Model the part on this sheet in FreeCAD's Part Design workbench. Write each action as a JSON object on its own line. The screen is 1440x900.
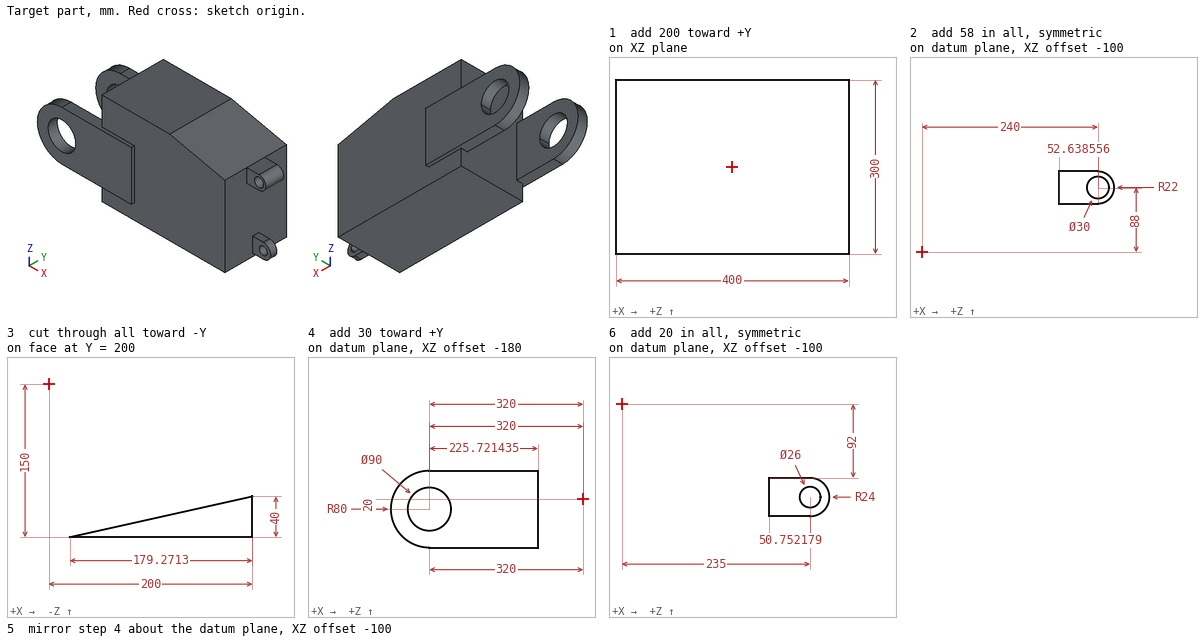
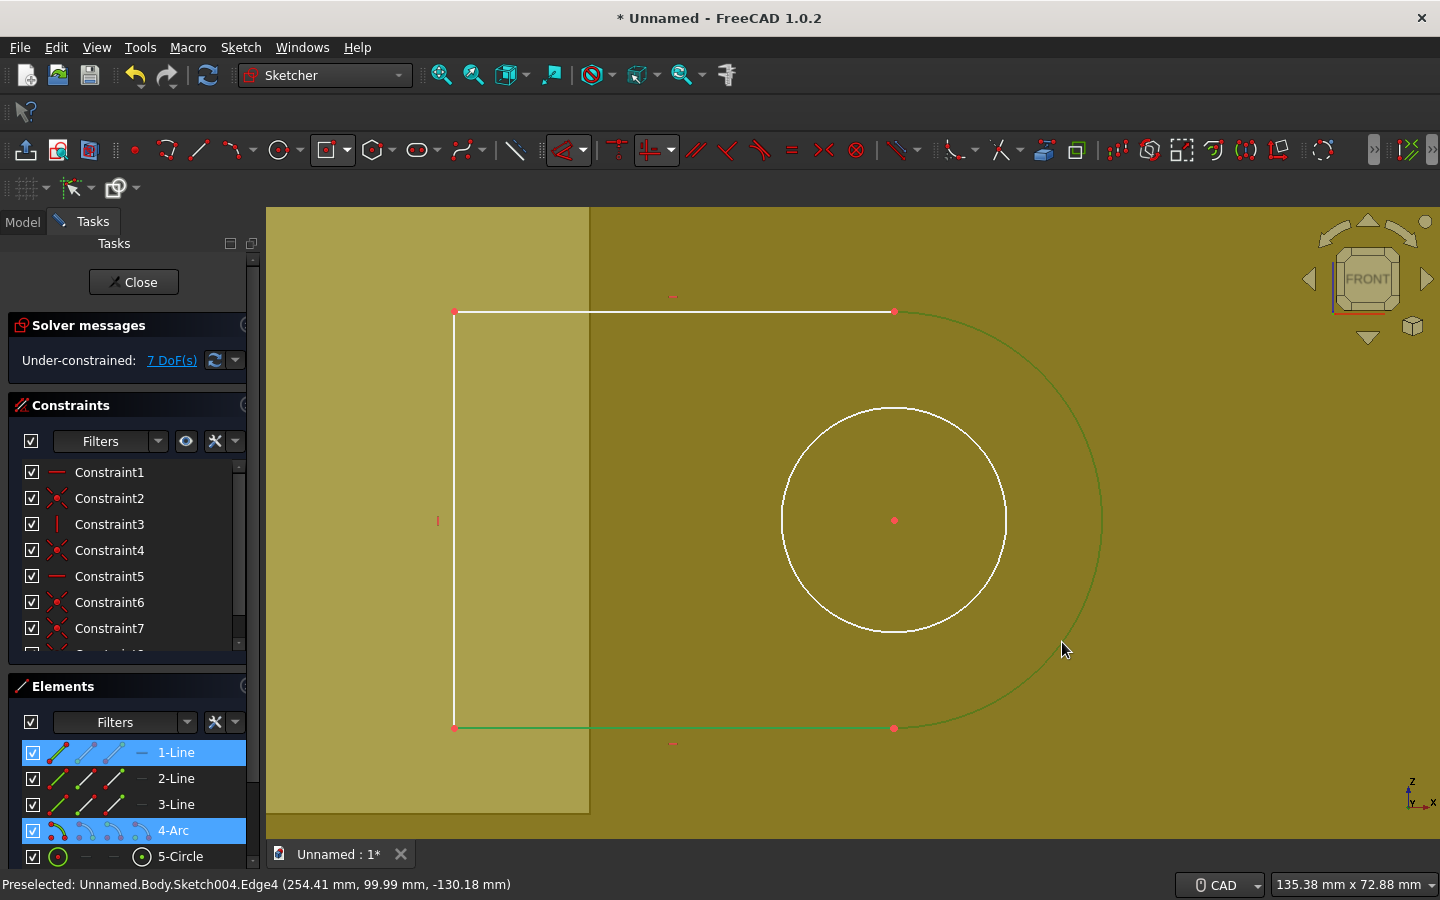
{"action": "left_click", "coordinate": [760, 150]}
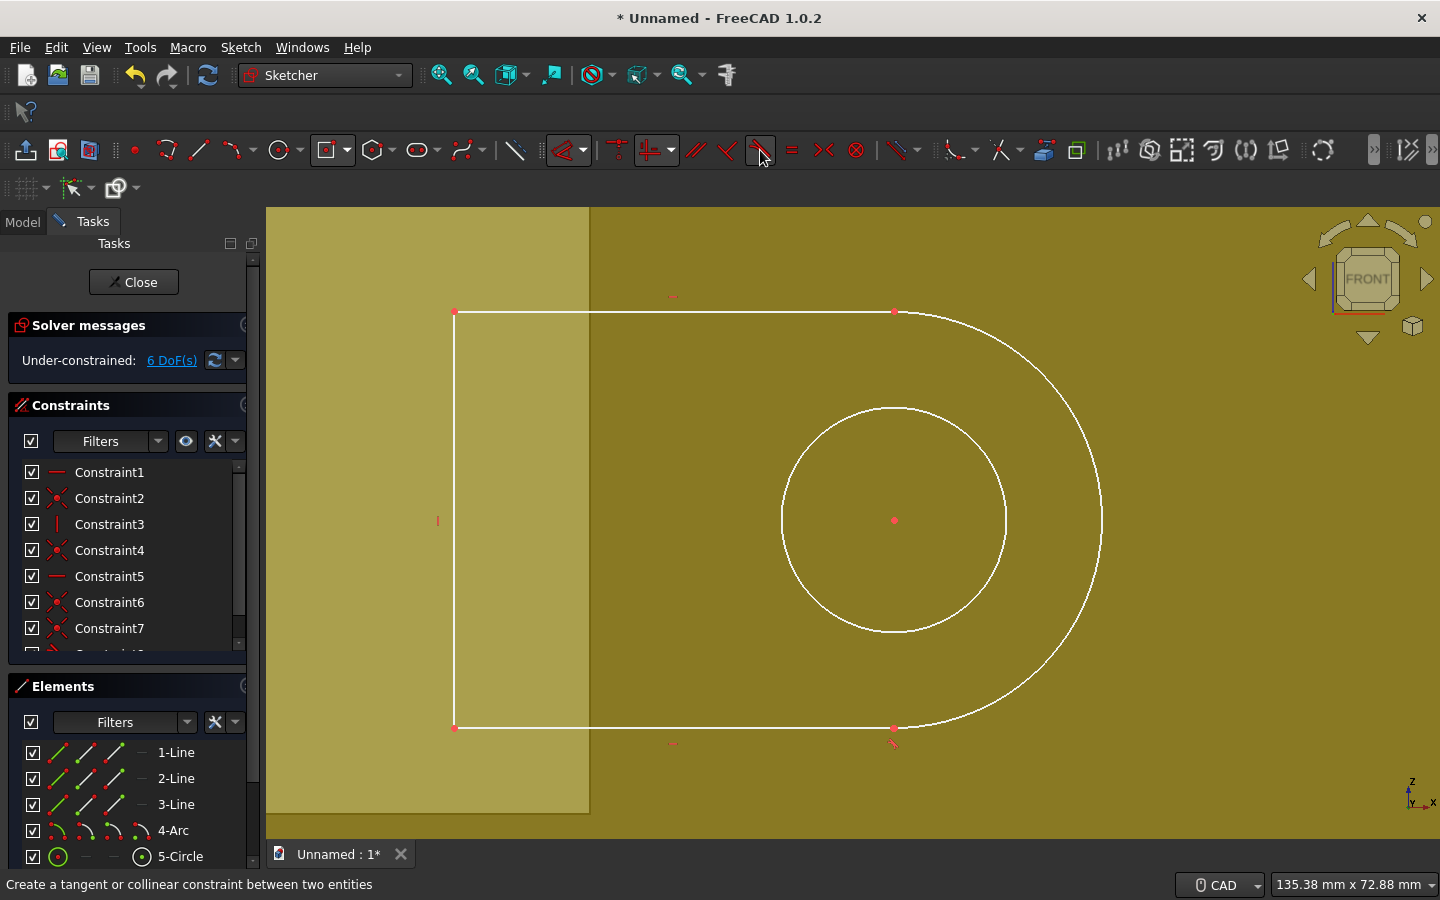
{"action": "left_click", "coordinate": [586, 312]}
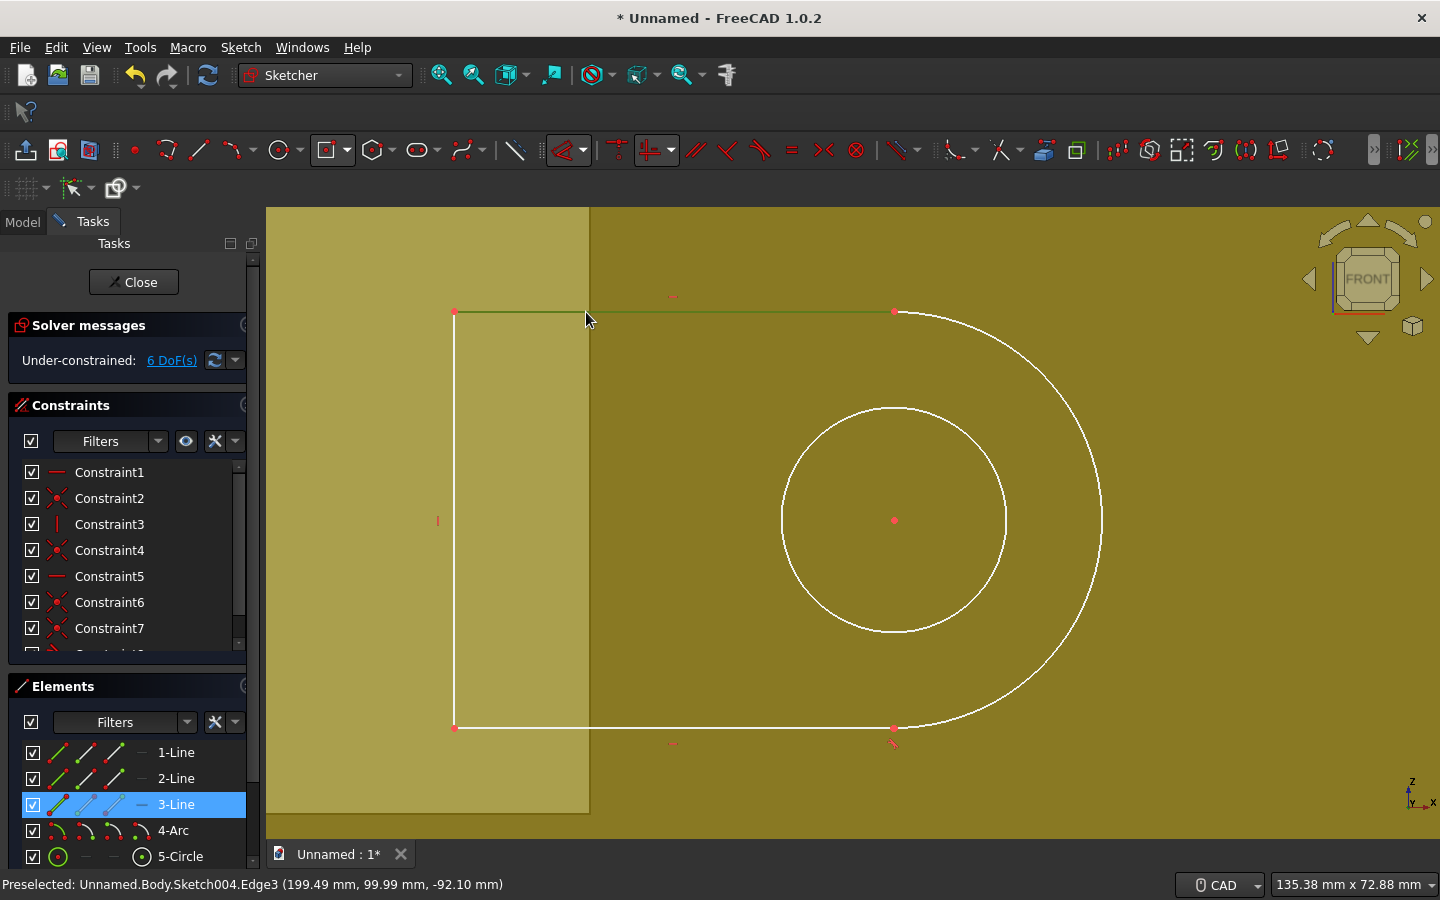
{"action": "left_click", "coordinate": [1062, 642]}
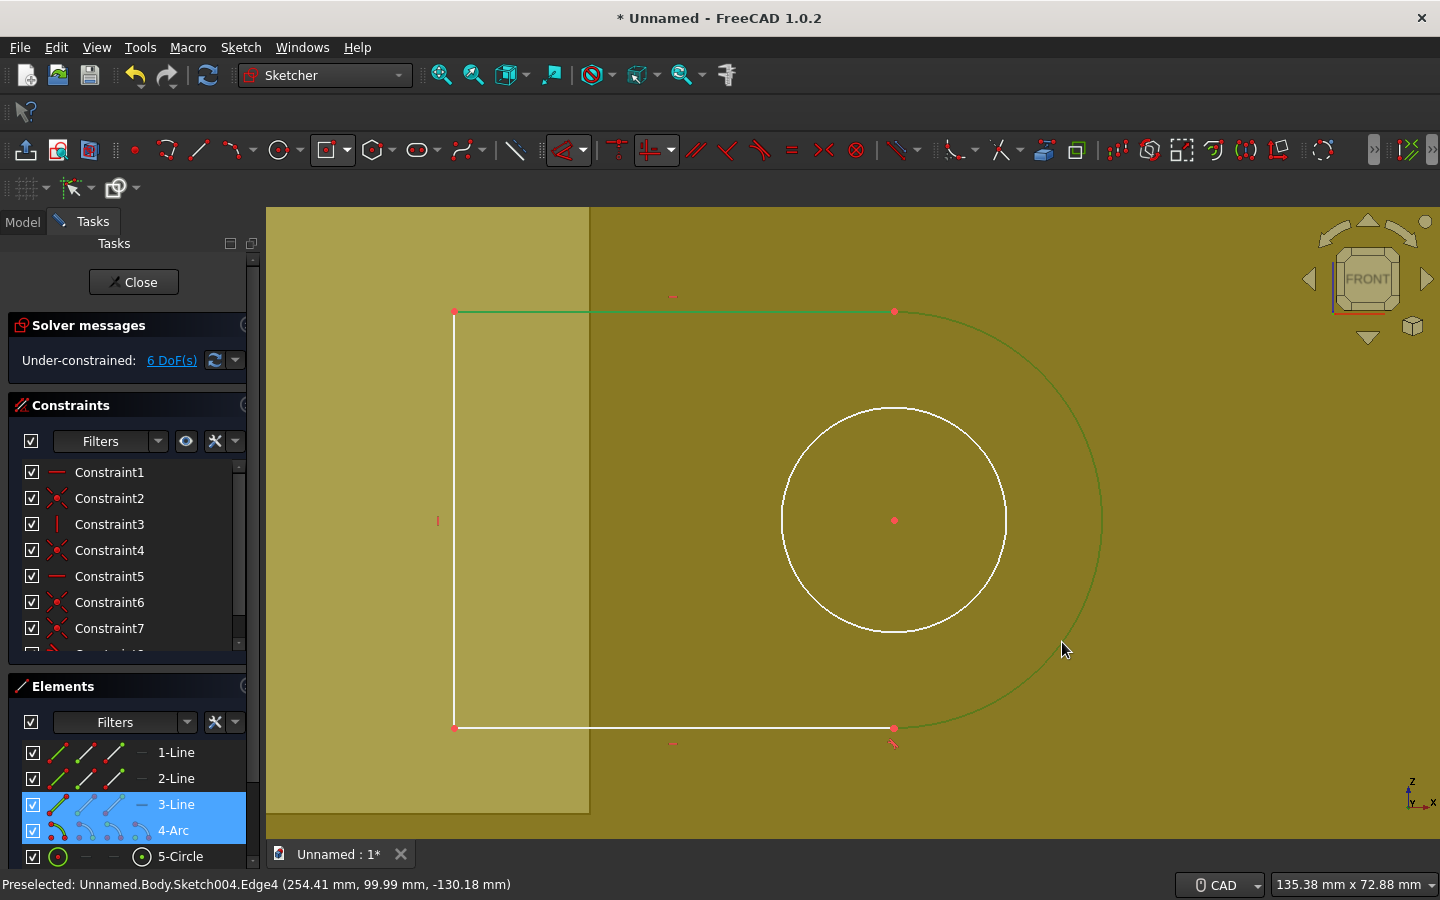
{"action": "left_click", "coordinate": [760, 150]}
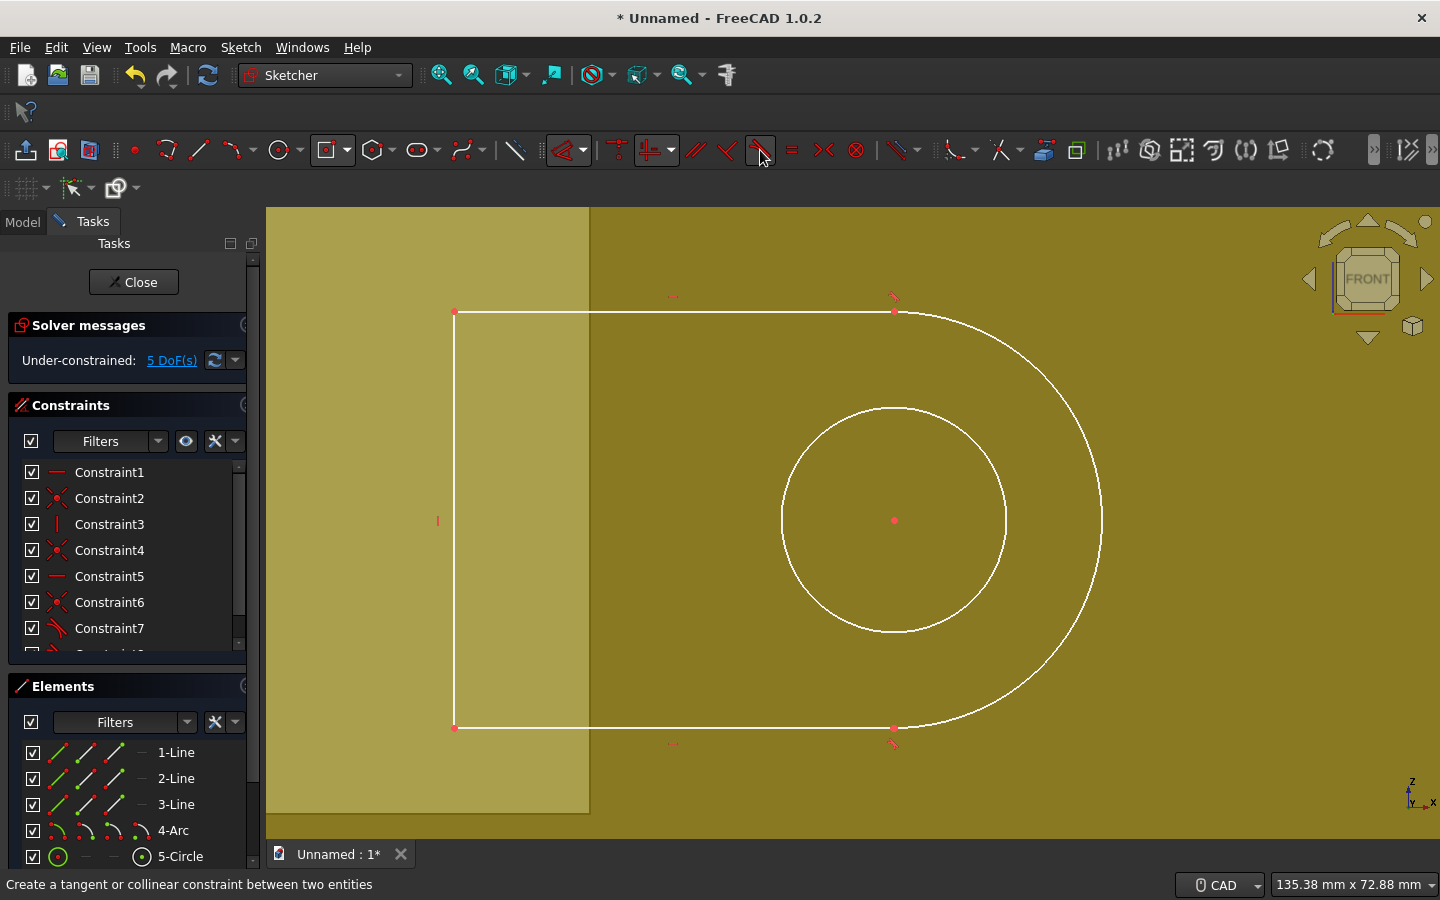
{"action": "left_click", "coordinate": [1062, 642]}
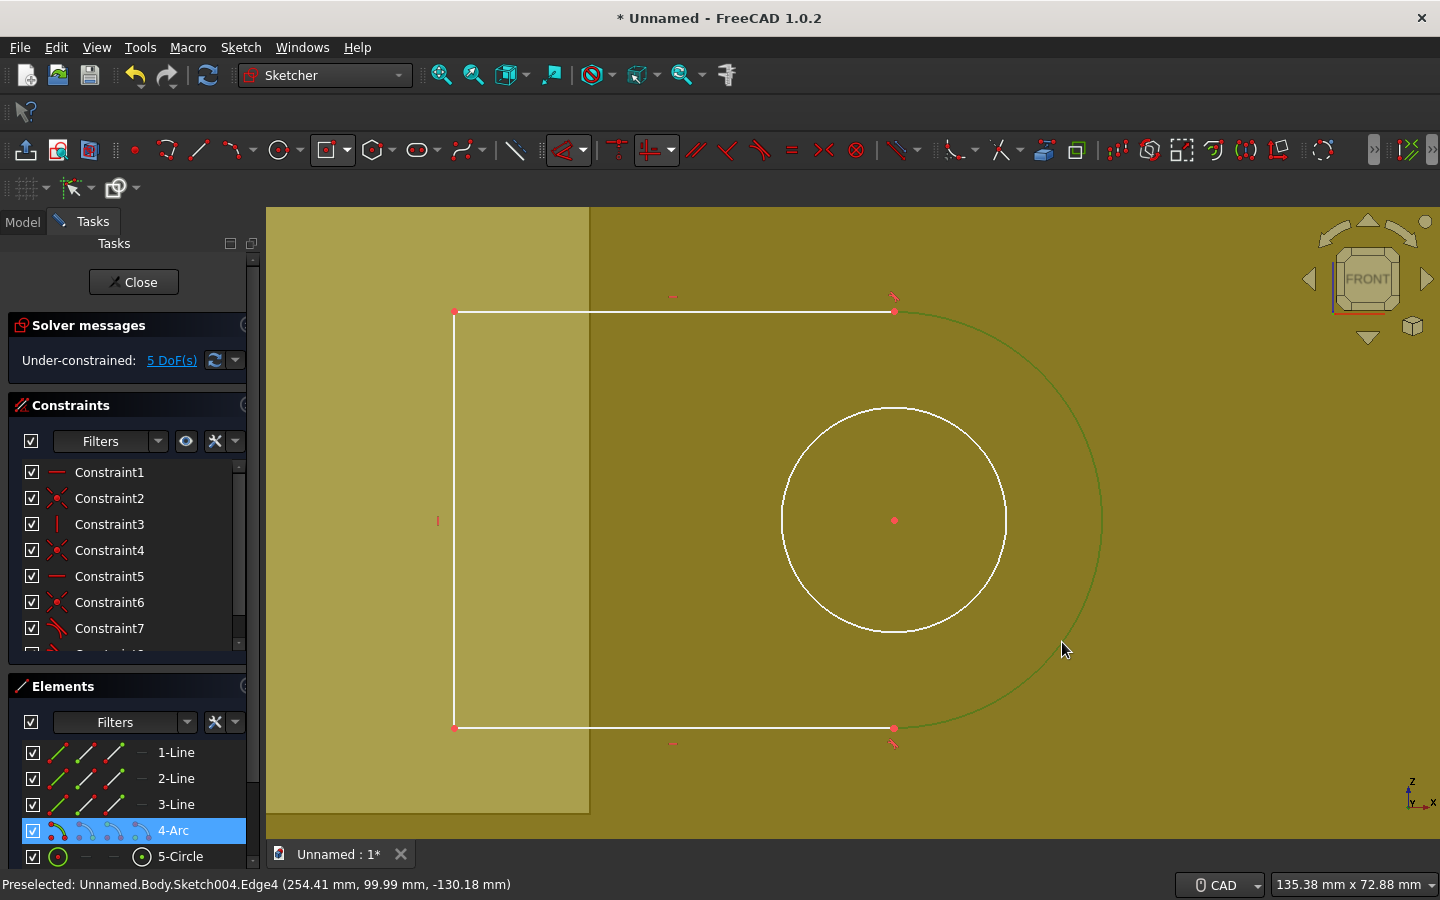
{"action": "left_click", "coordinate": [586, 150]}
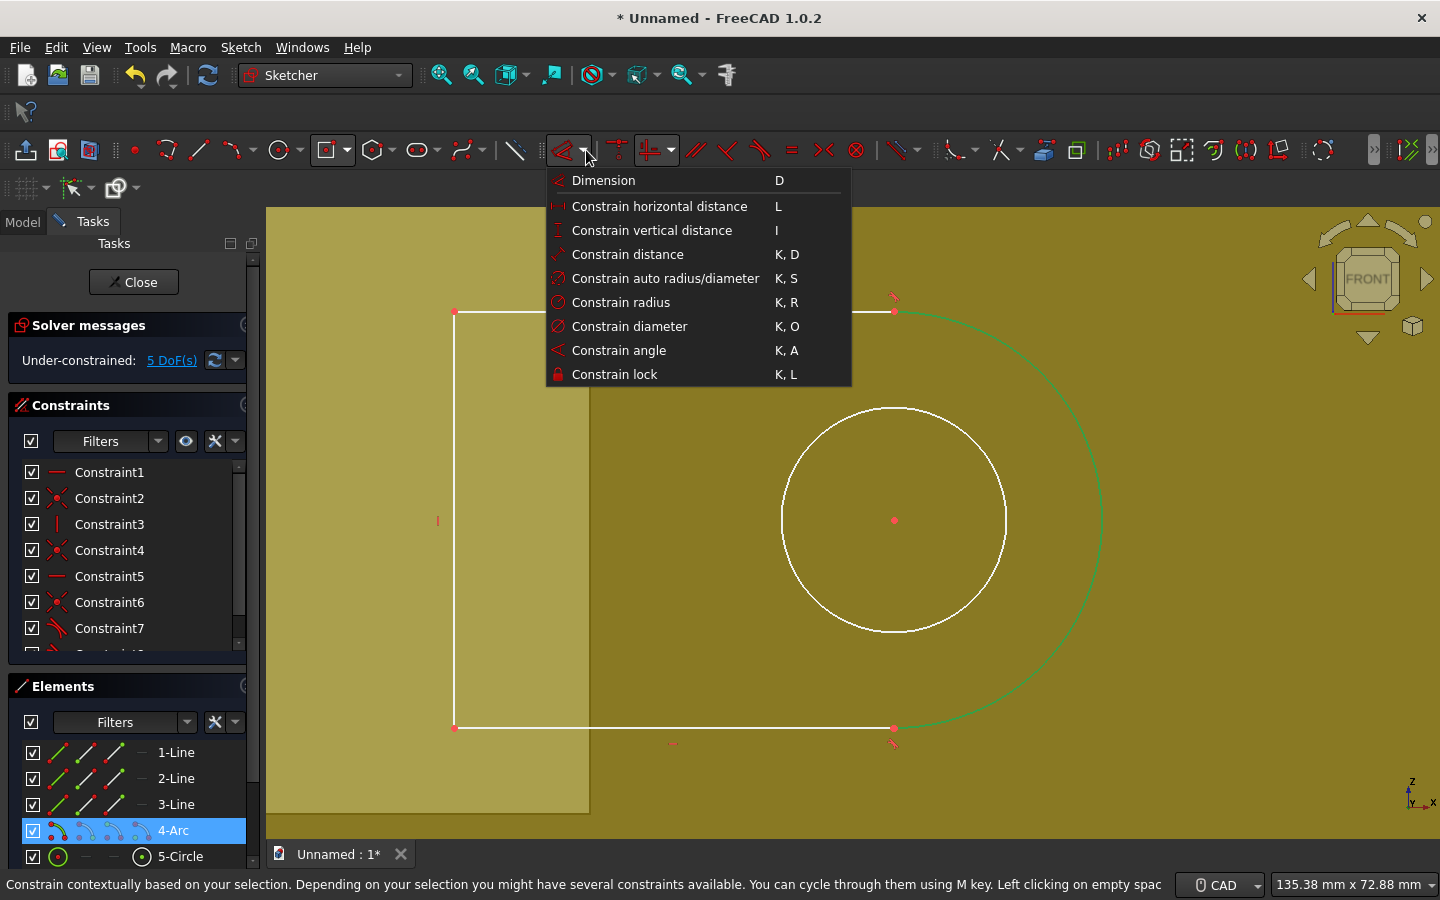
{"action": "left_click", "coordinate": [699, 302]}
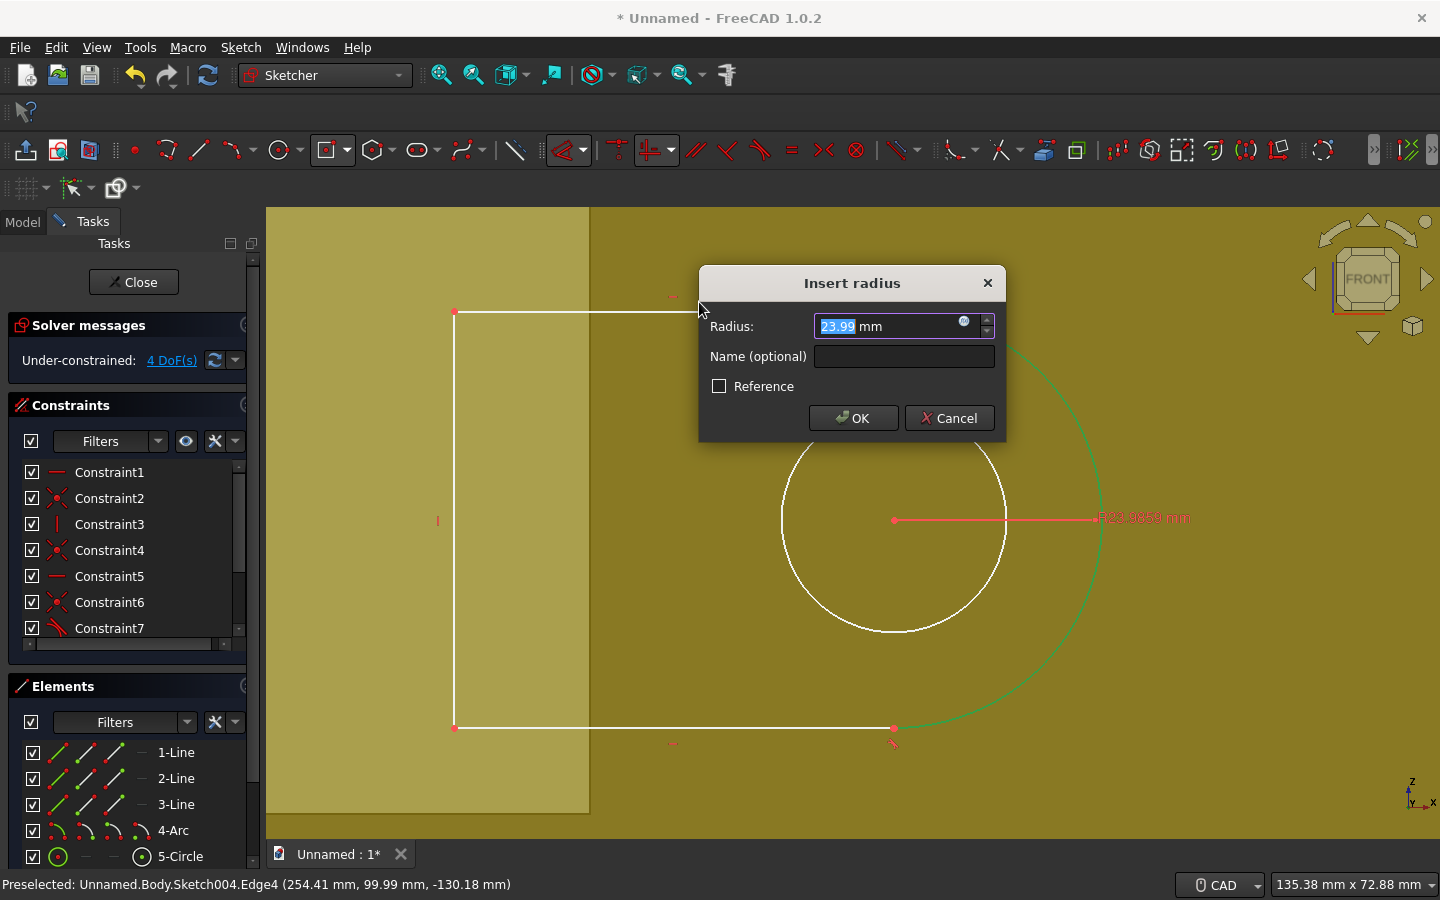
{"action": "type", "text": "24"}
{"action": "key", "text": "Return"}